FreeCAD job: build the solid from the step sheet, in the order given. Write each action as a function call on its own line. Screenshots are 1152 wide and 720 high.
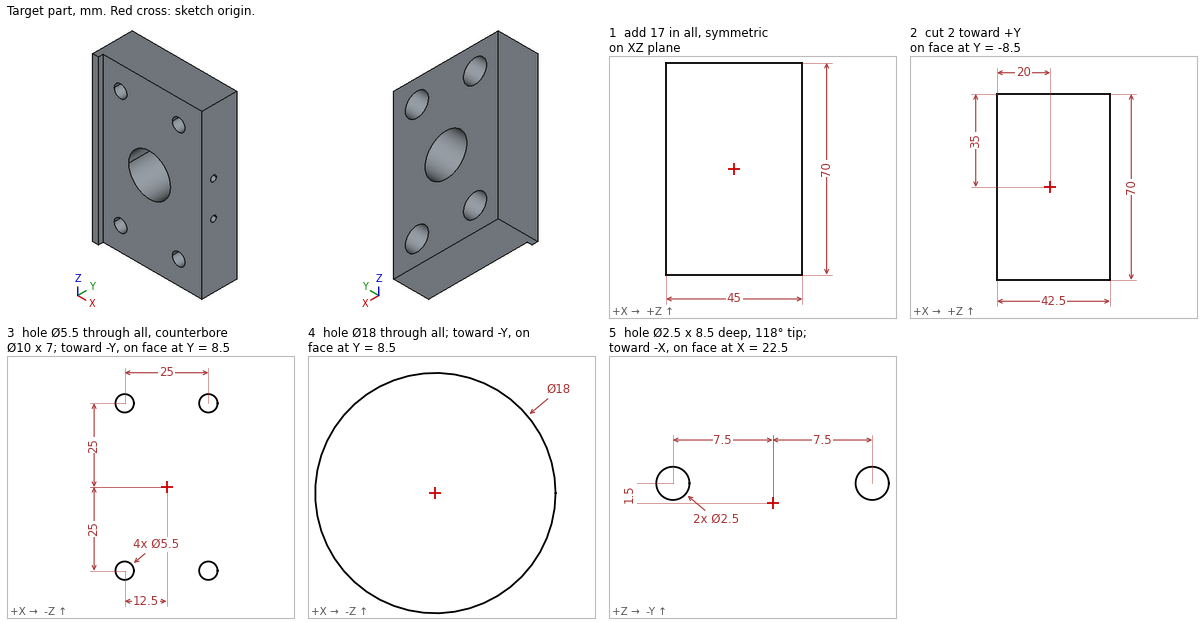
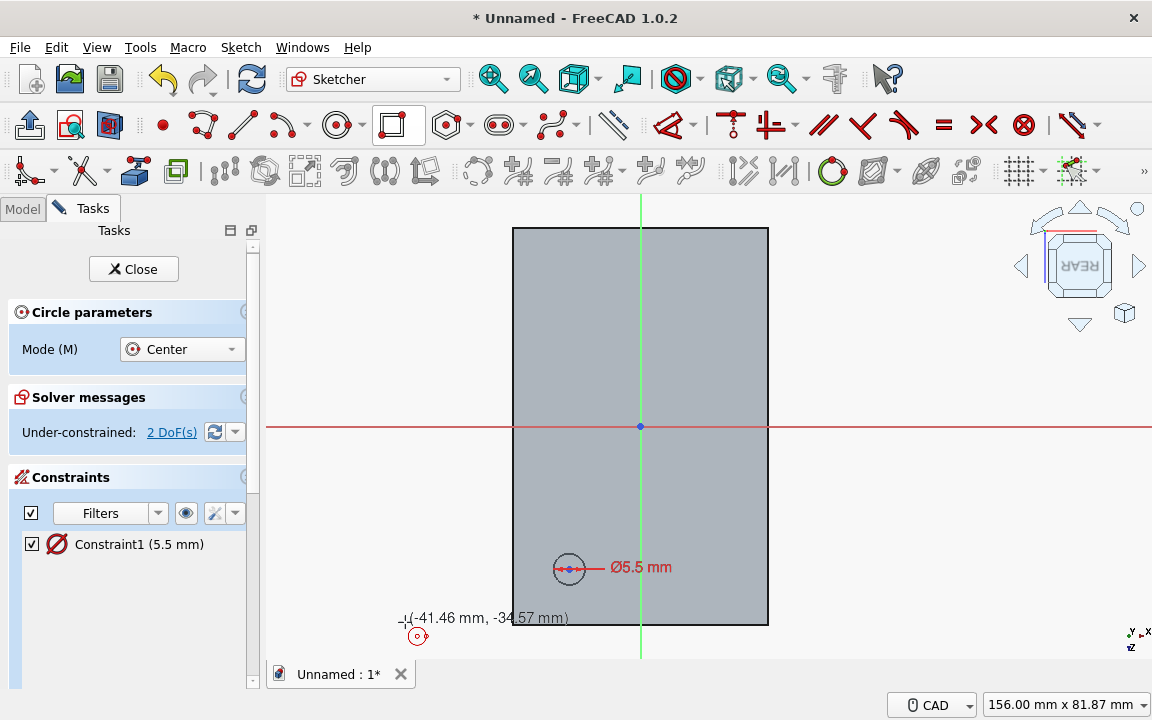
scroll(570, 285, up, 2)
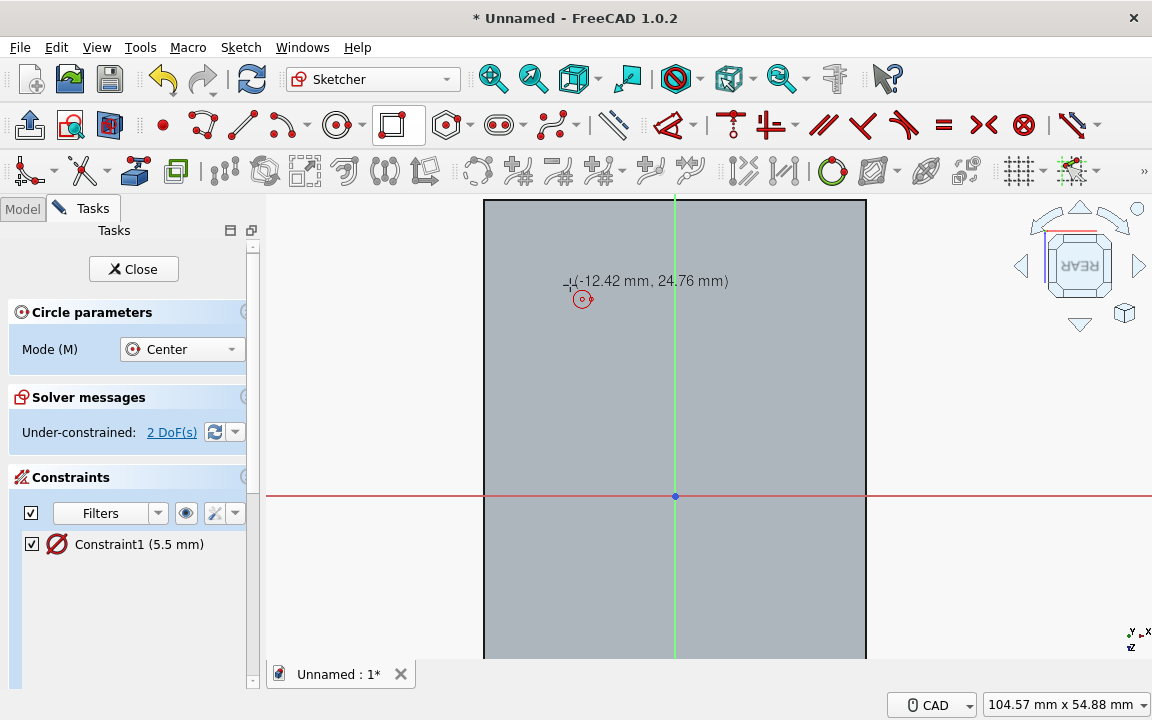
click(569, 284)
move(586, 268)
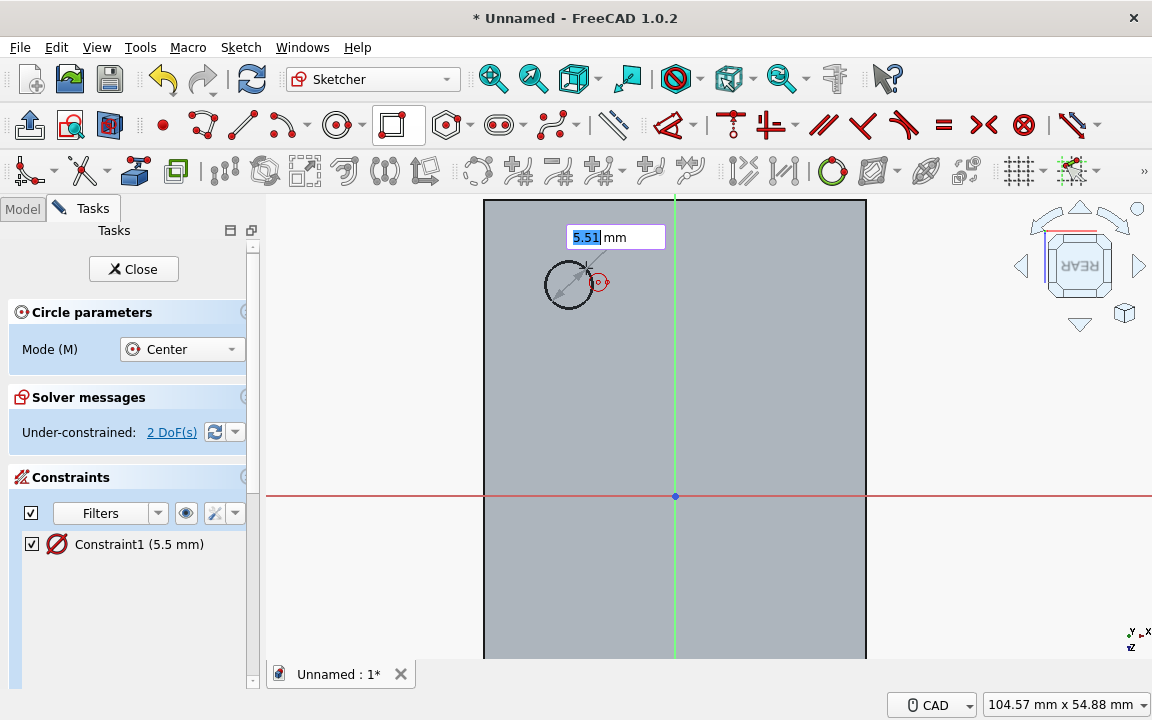
text(5.5)
key(Return)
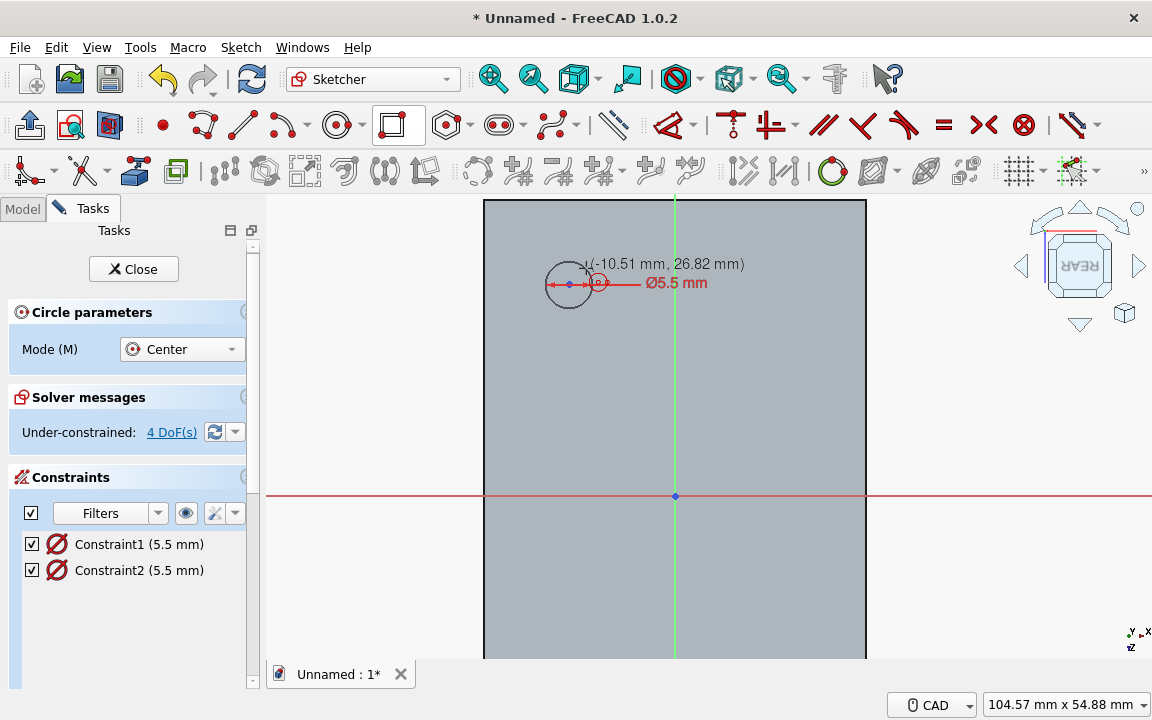
click(781, 284)
move(797, 268)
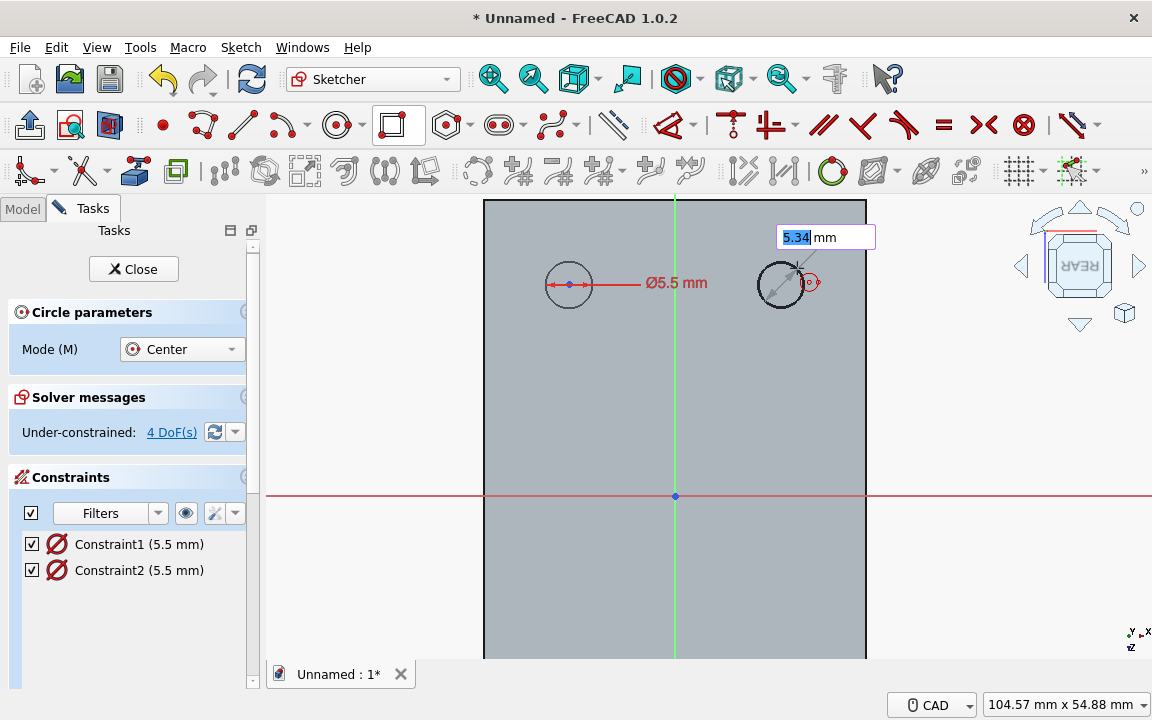
text(5.5)
key(Return)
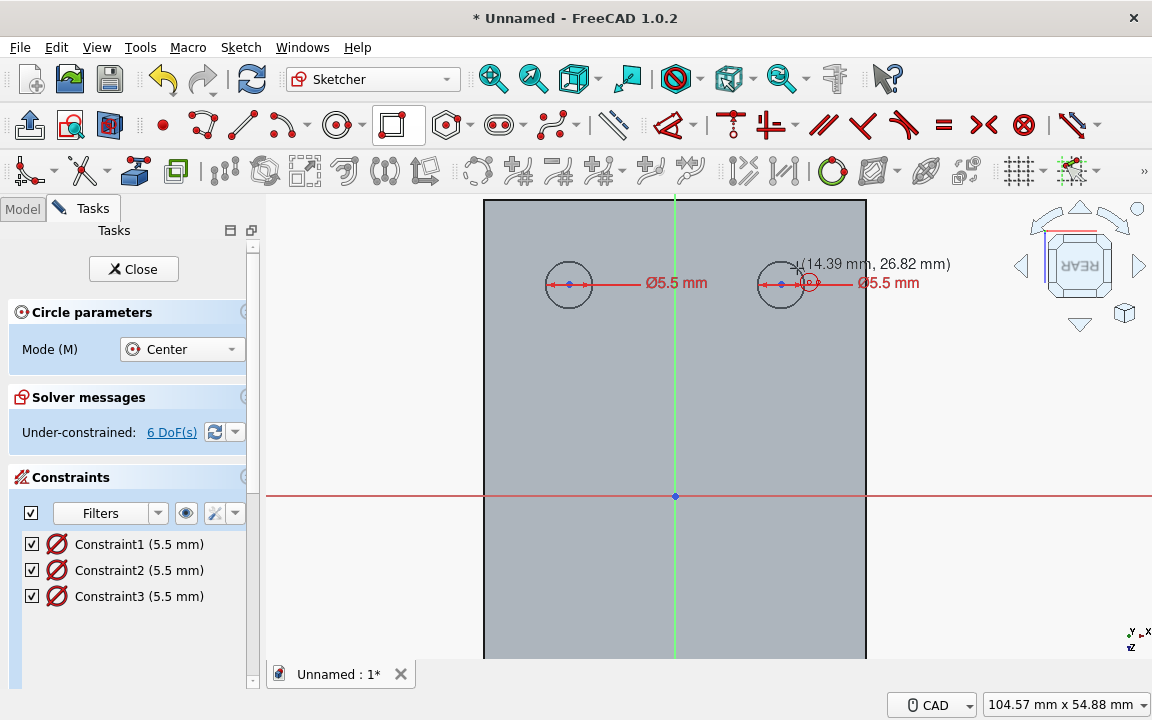
scroll(570, 285, down, 2)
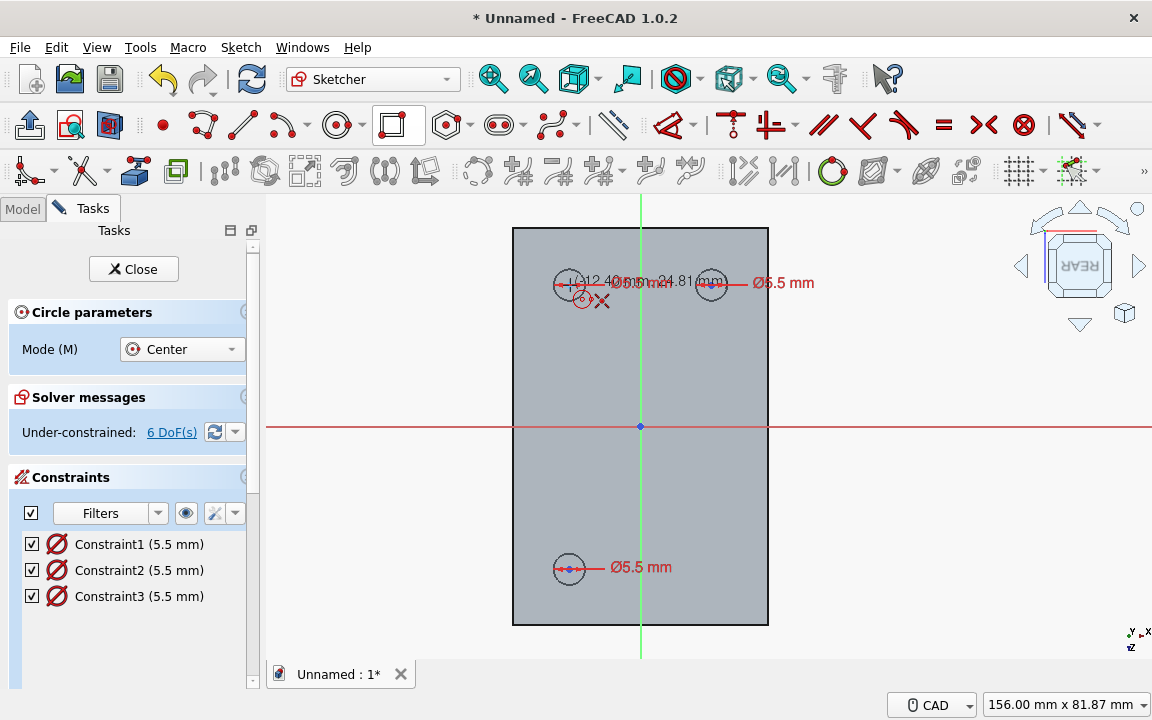
scroll(712, 569, up, 2)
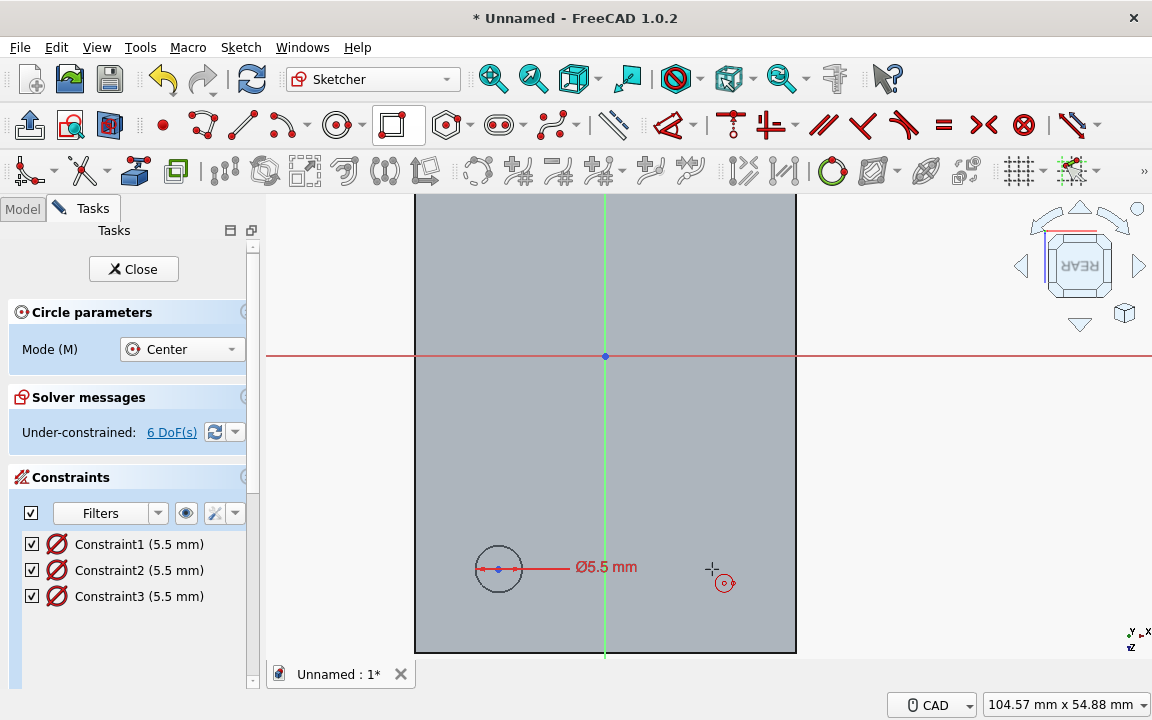
click(711, 568)
move(728, 552)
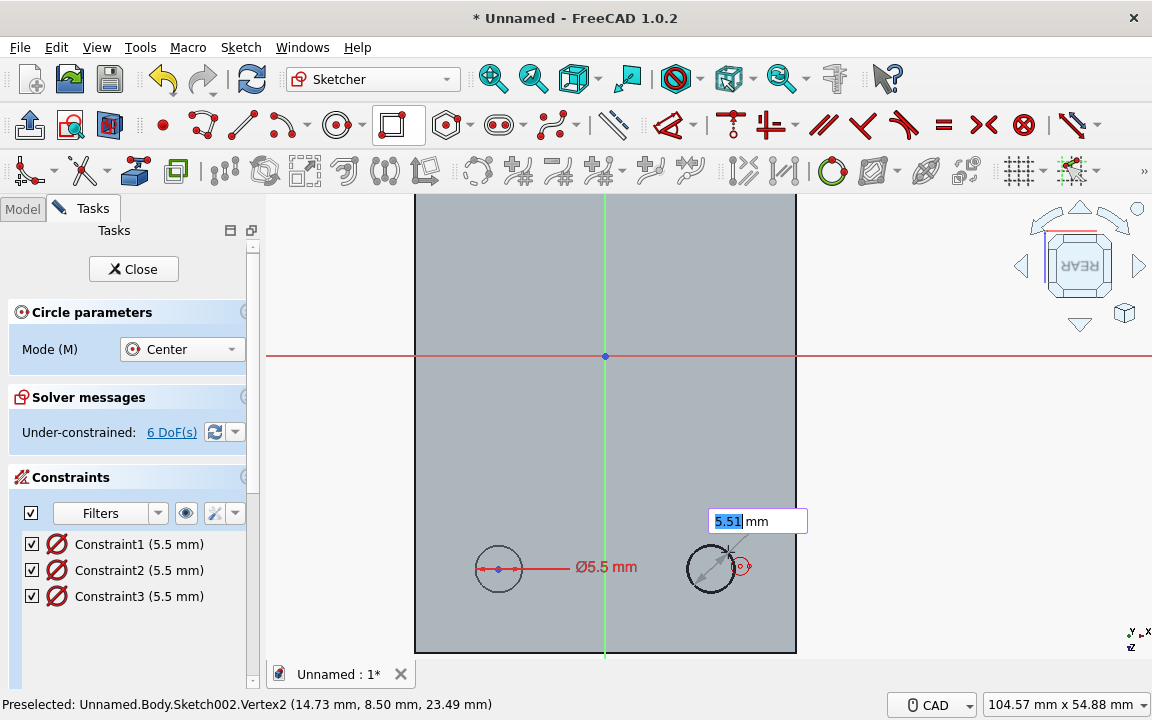
text(5.5)
key(Return)
key(Escape)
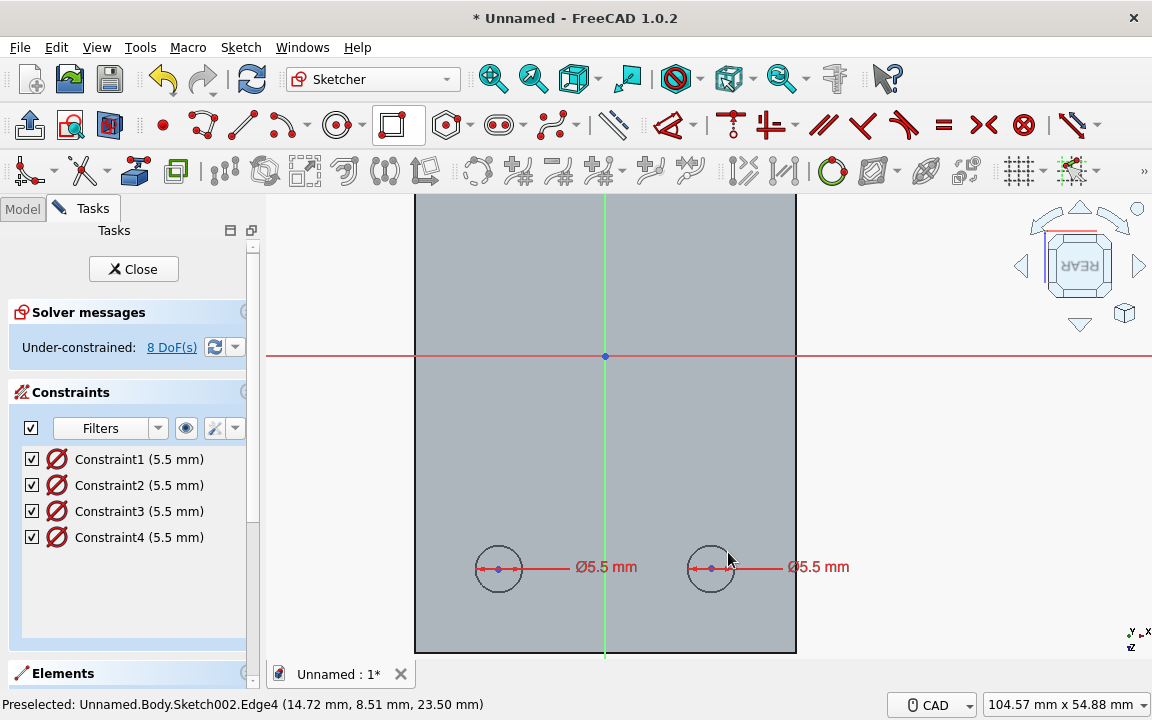
click(499, 569)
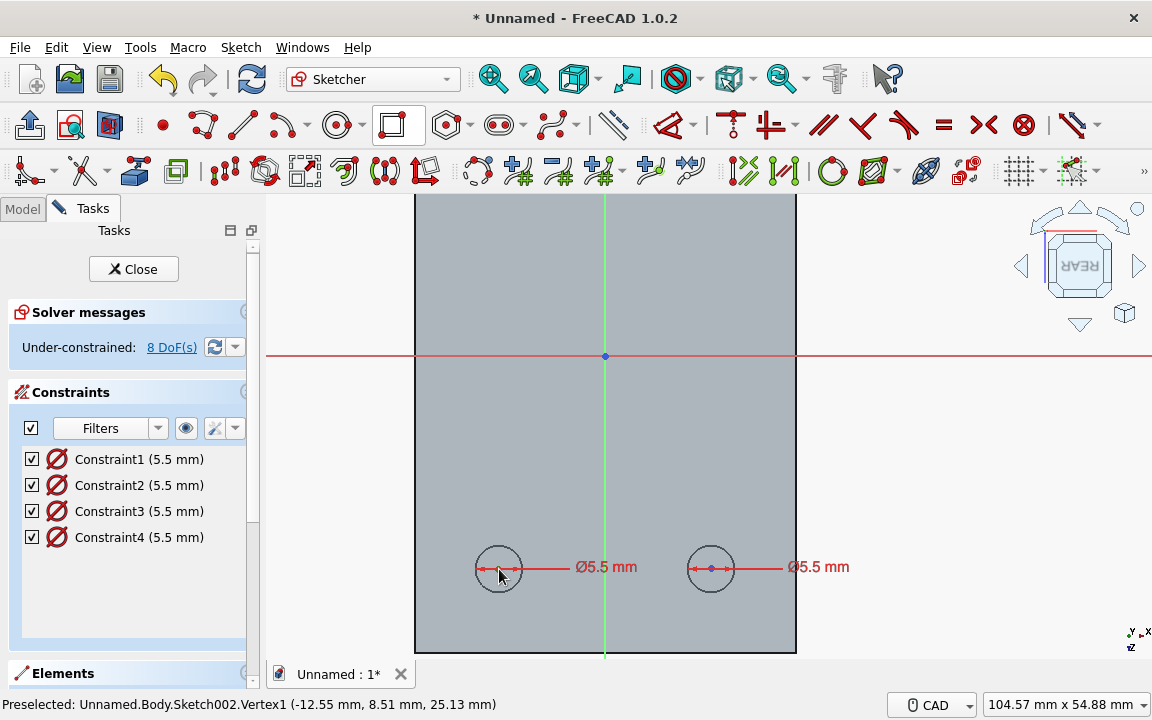
scroll(712, 569, down, 2)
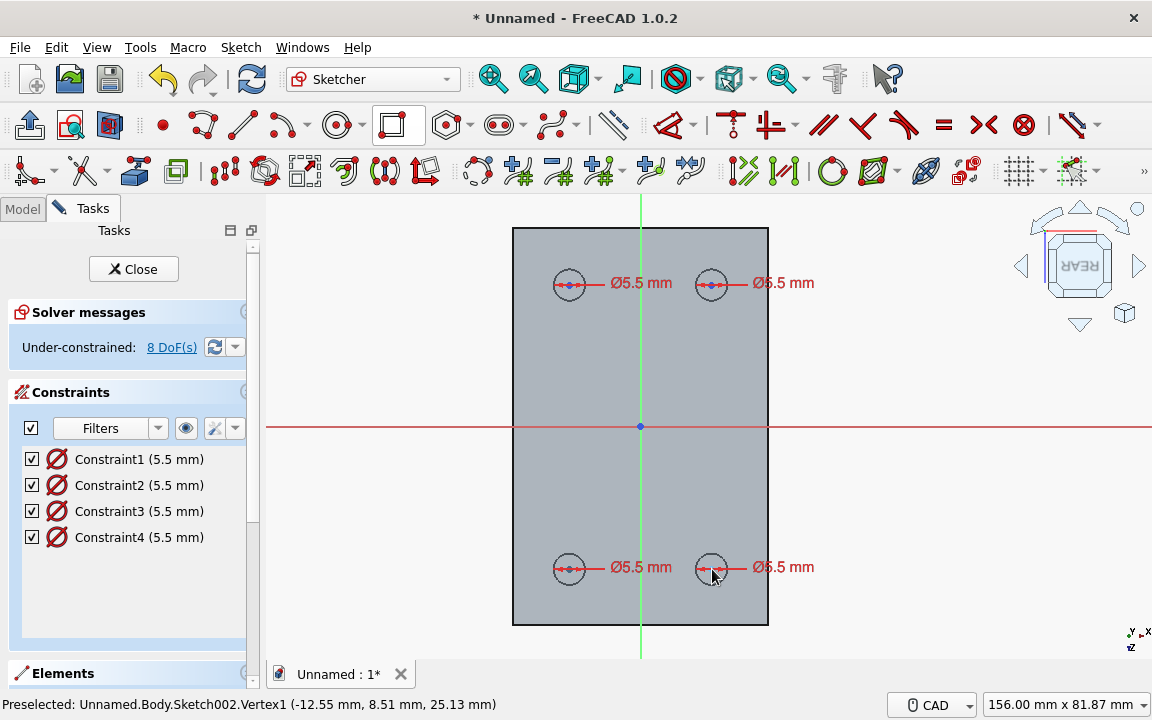
click(569, 285)